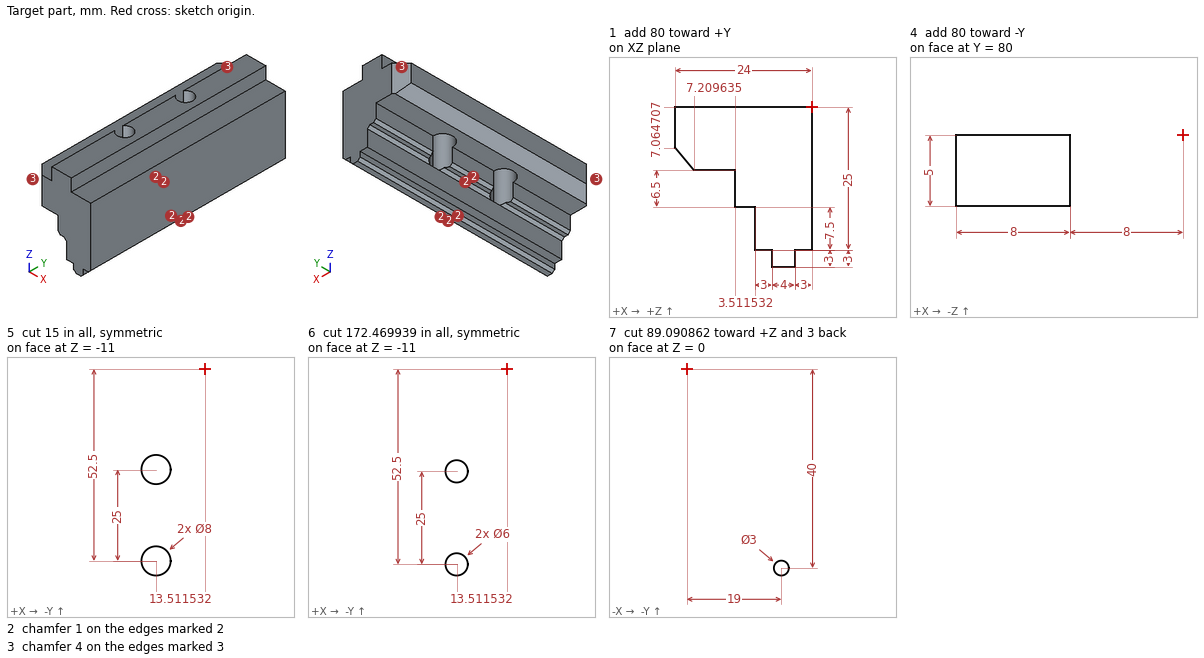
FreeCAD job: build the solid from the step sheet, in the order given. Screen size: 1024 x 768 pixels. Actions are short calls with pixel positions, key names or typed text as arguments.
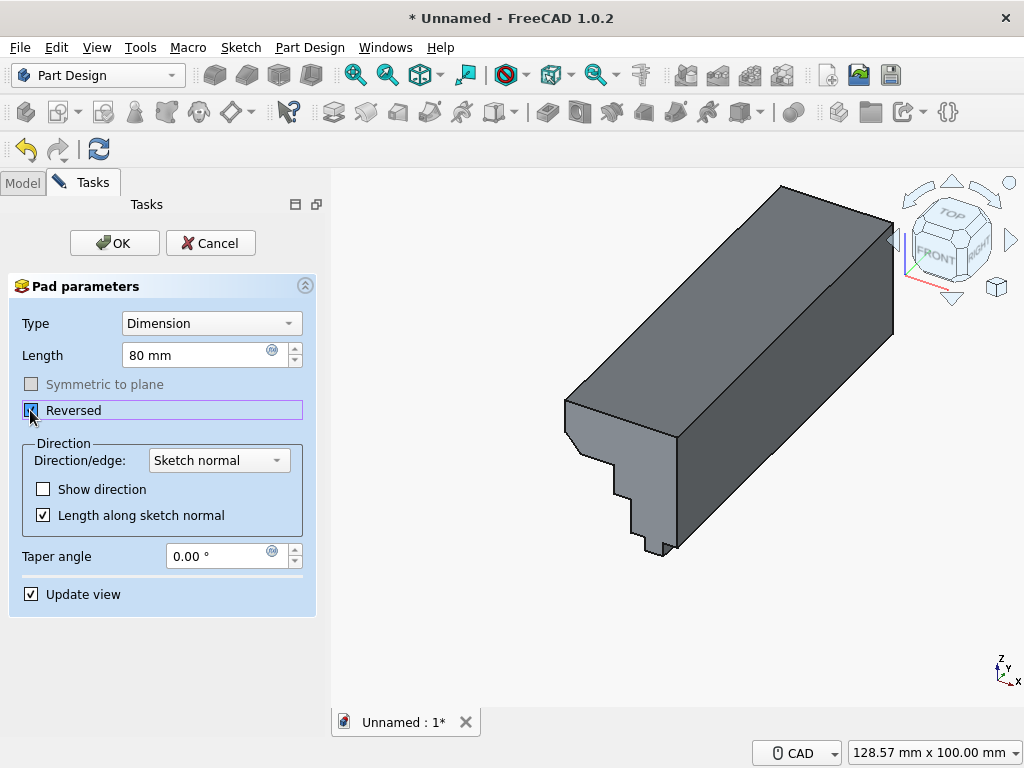
click(115, 243)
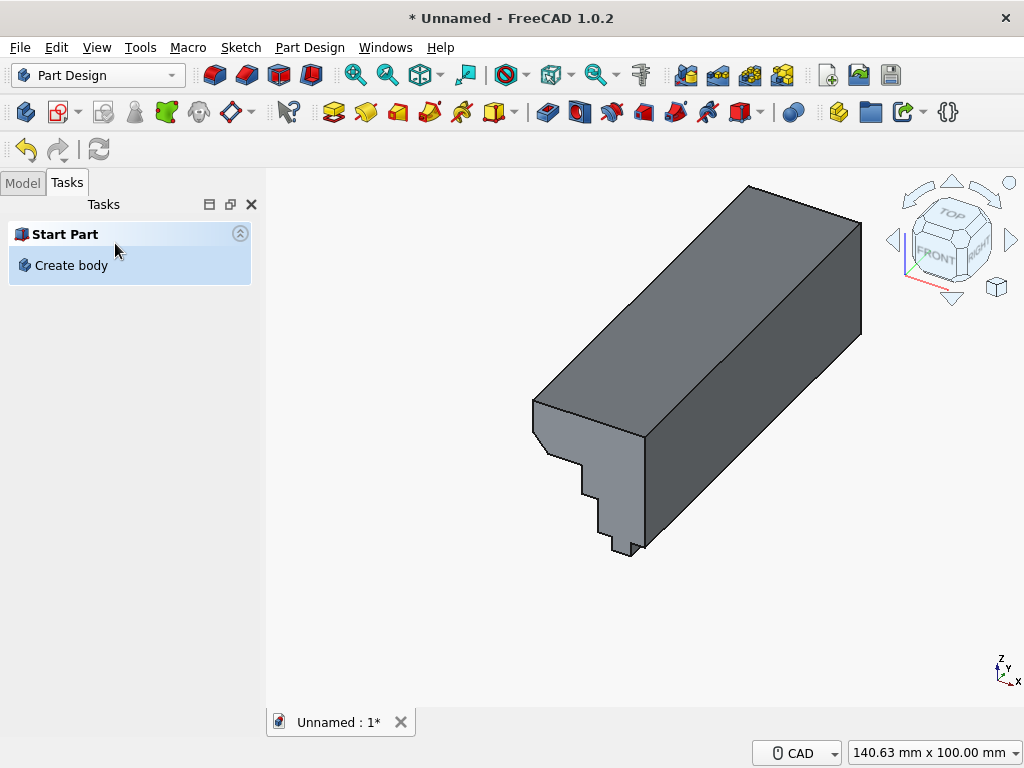
key(0)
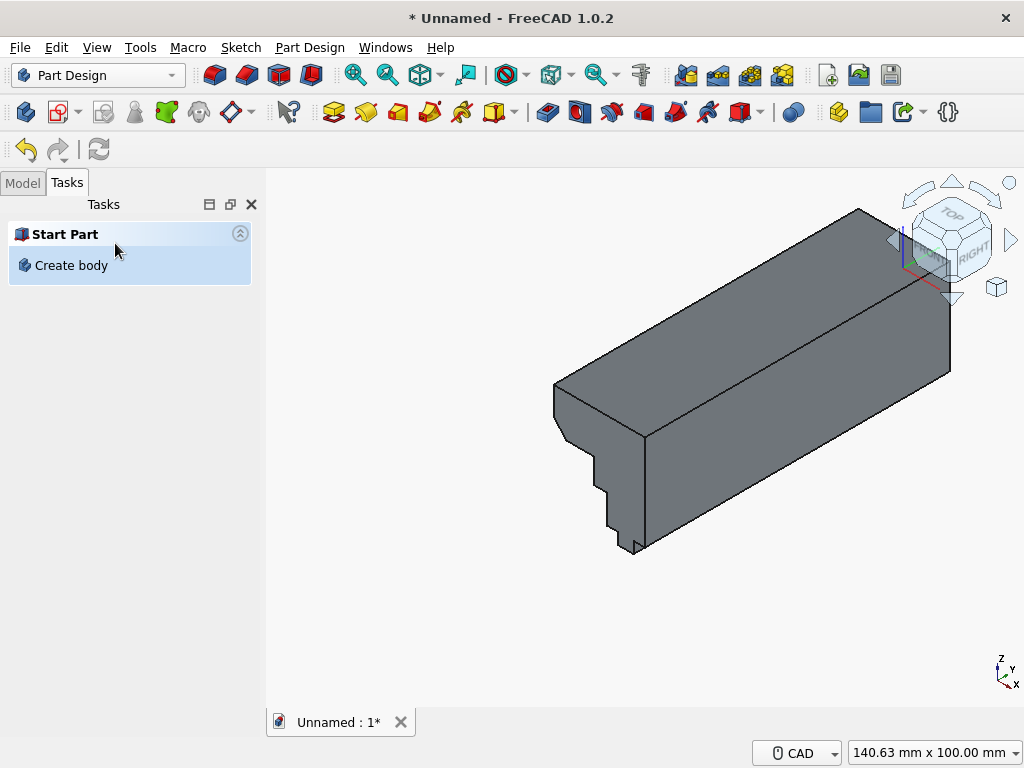
key(2)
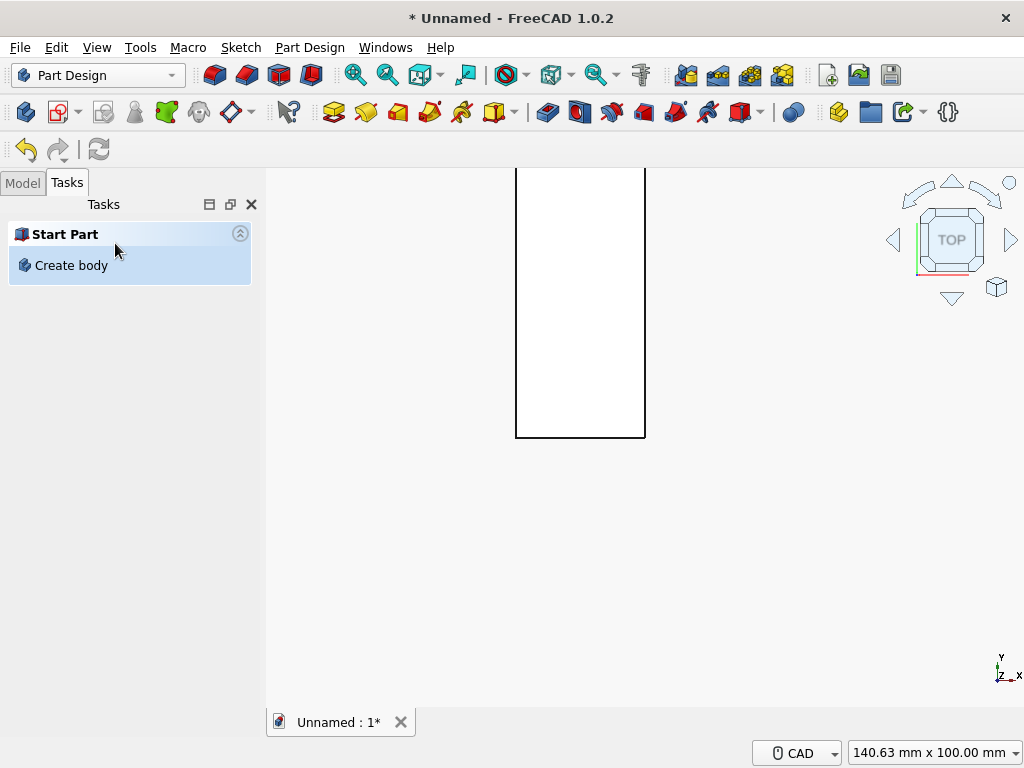
key(v)
key(f)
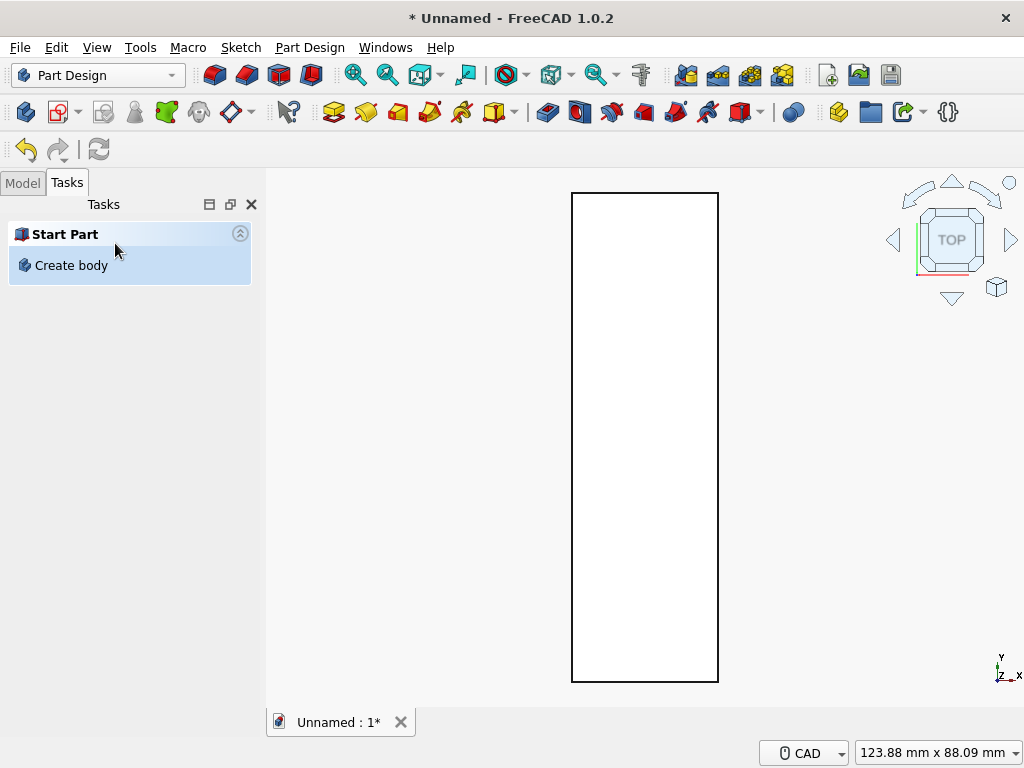
key(1)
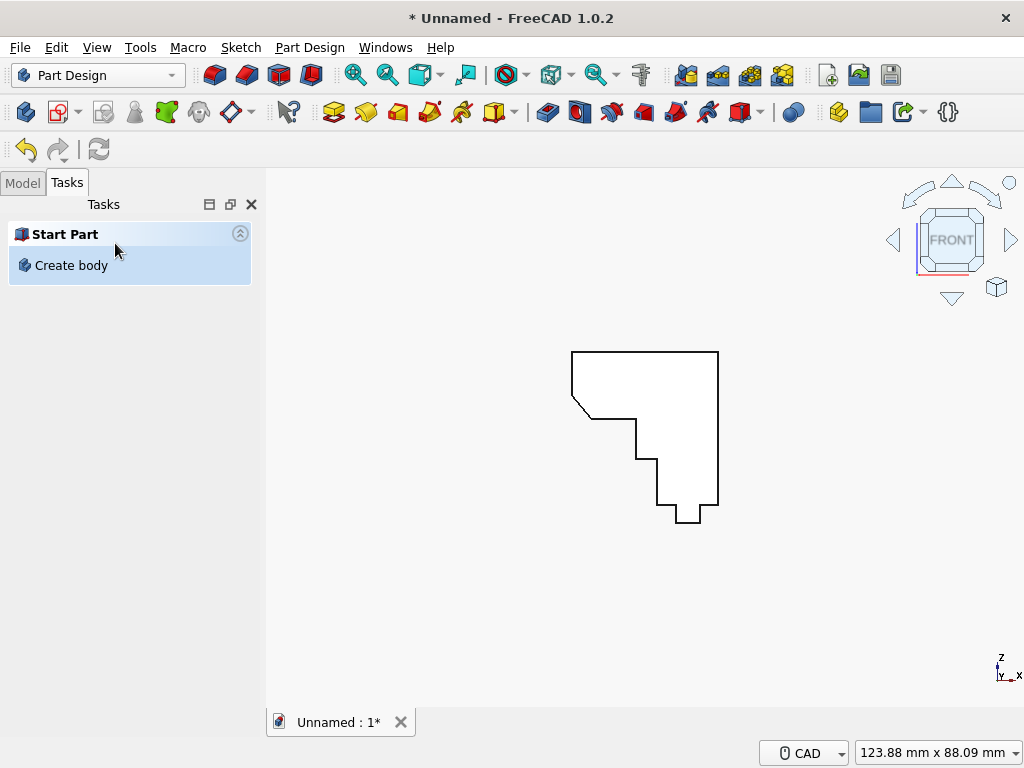
click(356, 76)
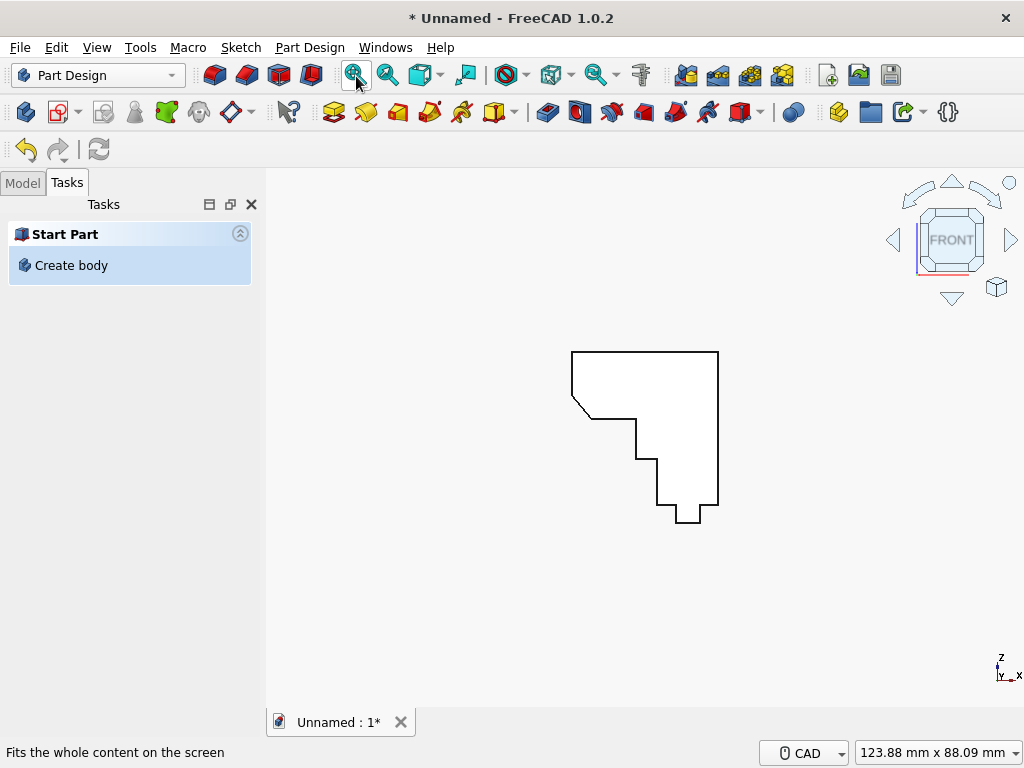
key(3)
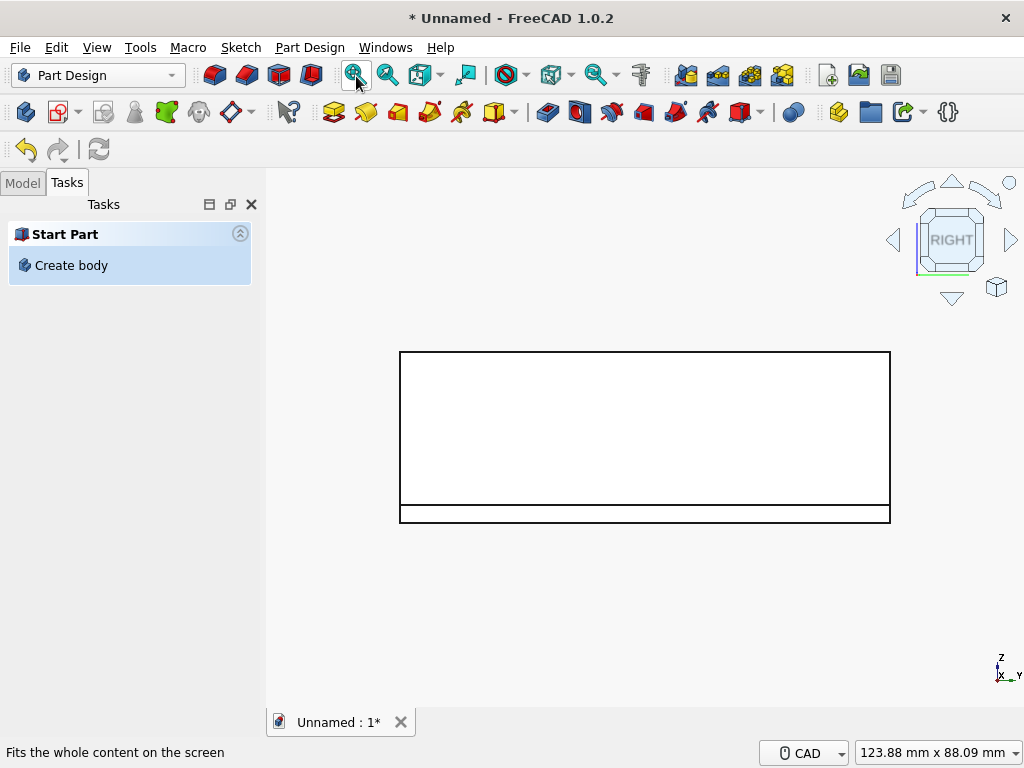
click(645, 522)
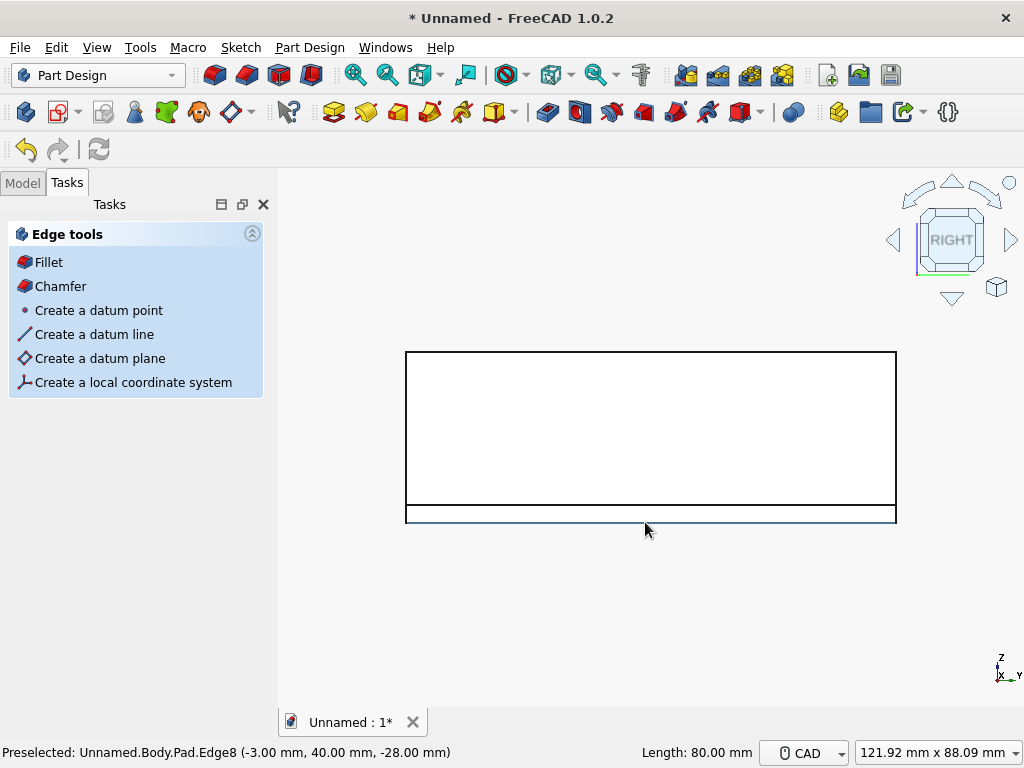
click(651, 504, ctrl)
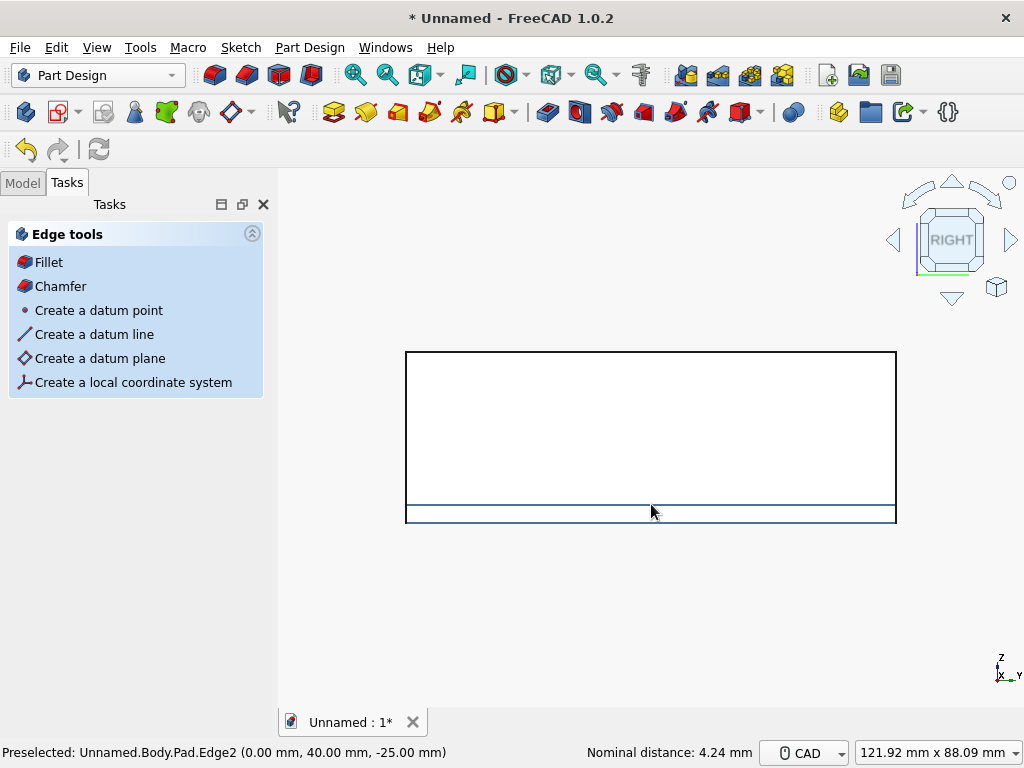
key(5)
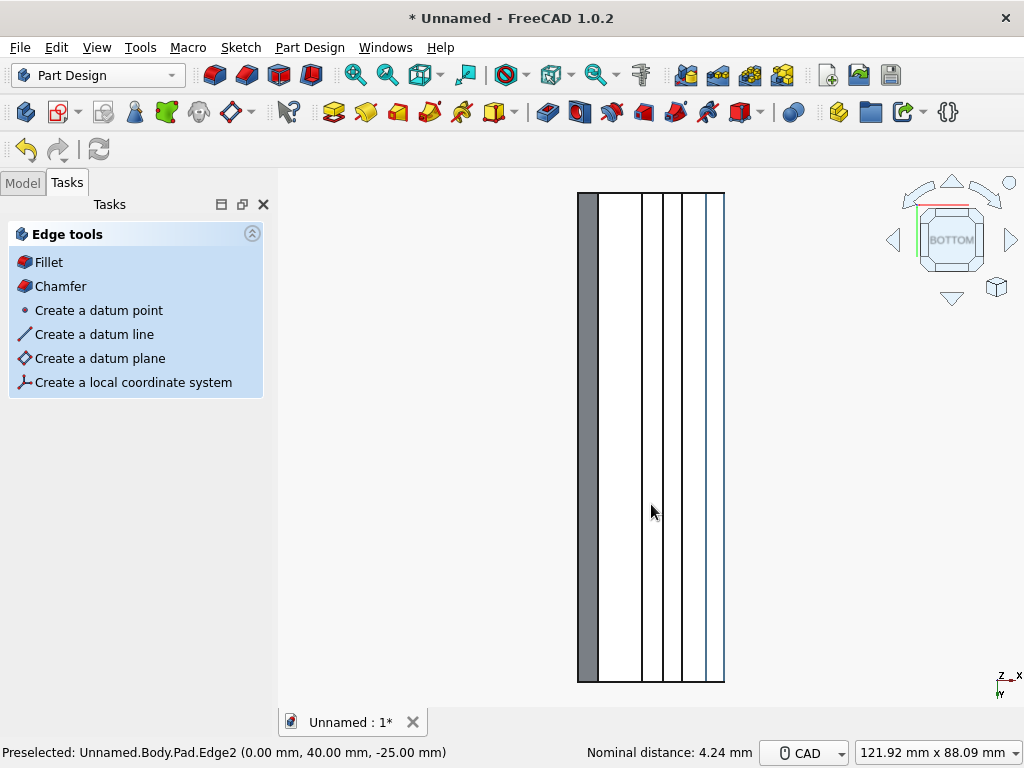
click(642, 436, ctrl)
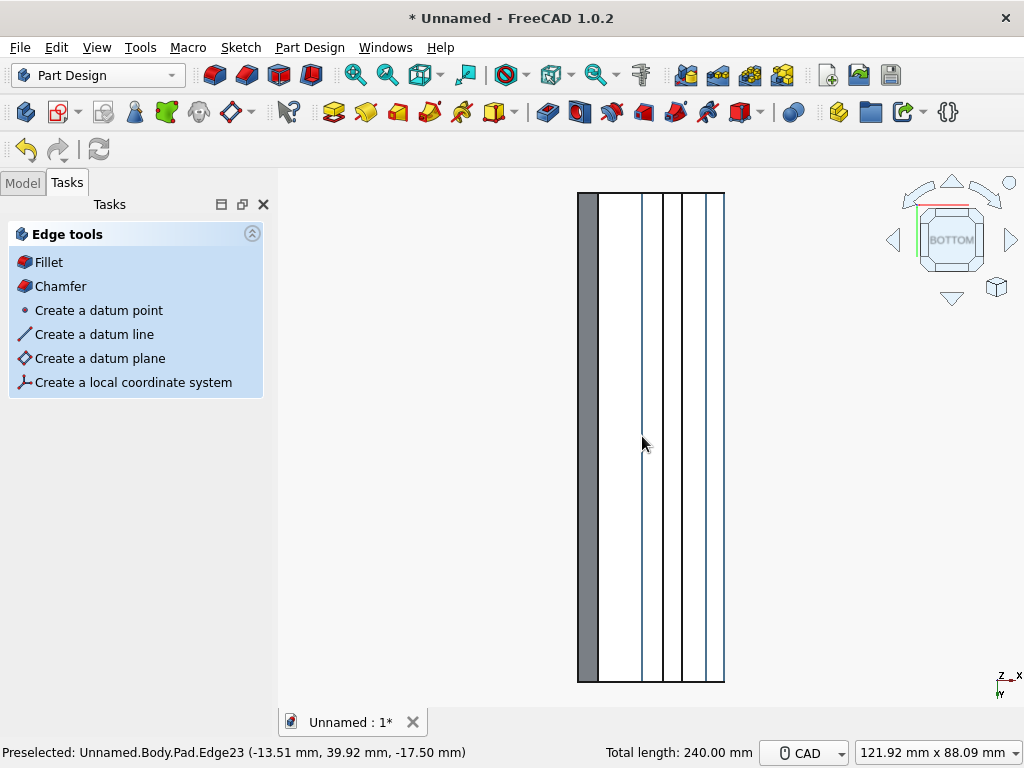
click(682, 436, ctrl)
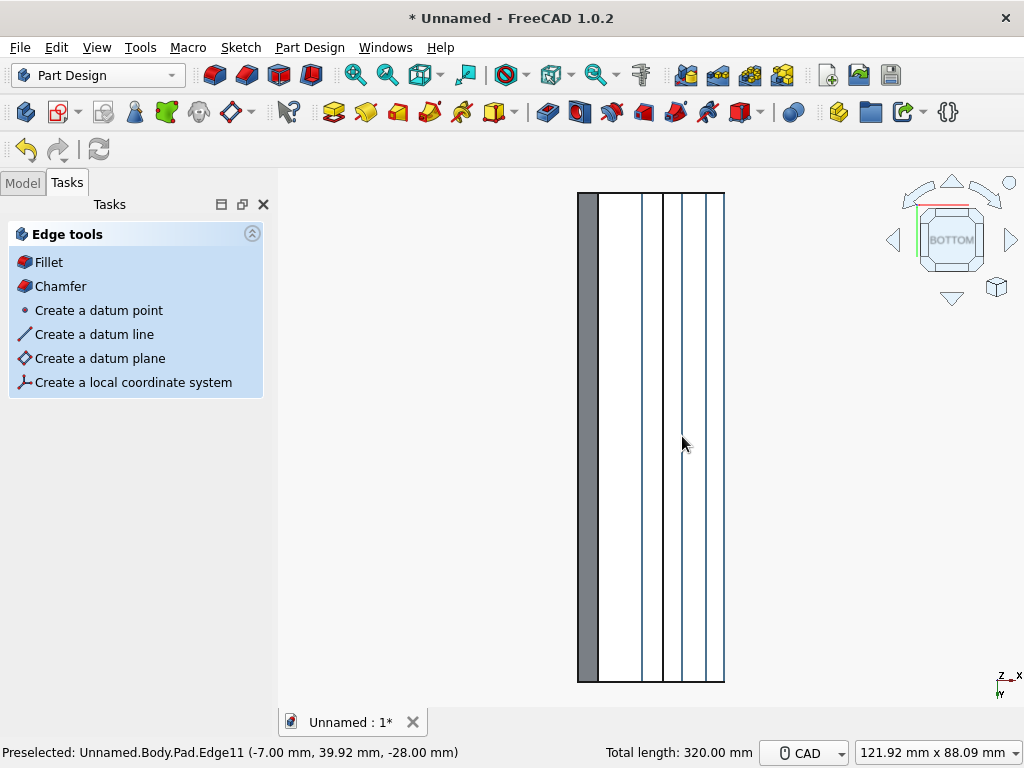
key(4)